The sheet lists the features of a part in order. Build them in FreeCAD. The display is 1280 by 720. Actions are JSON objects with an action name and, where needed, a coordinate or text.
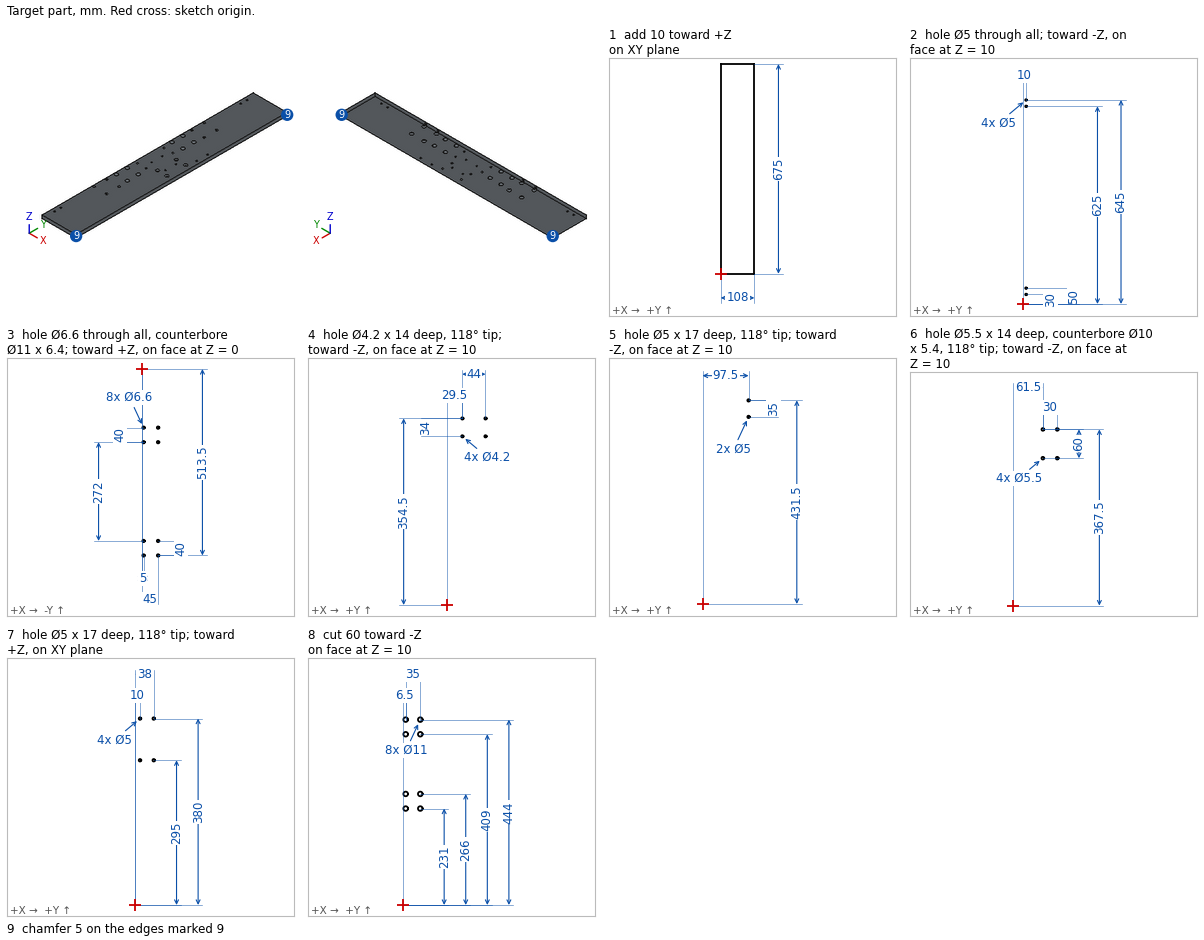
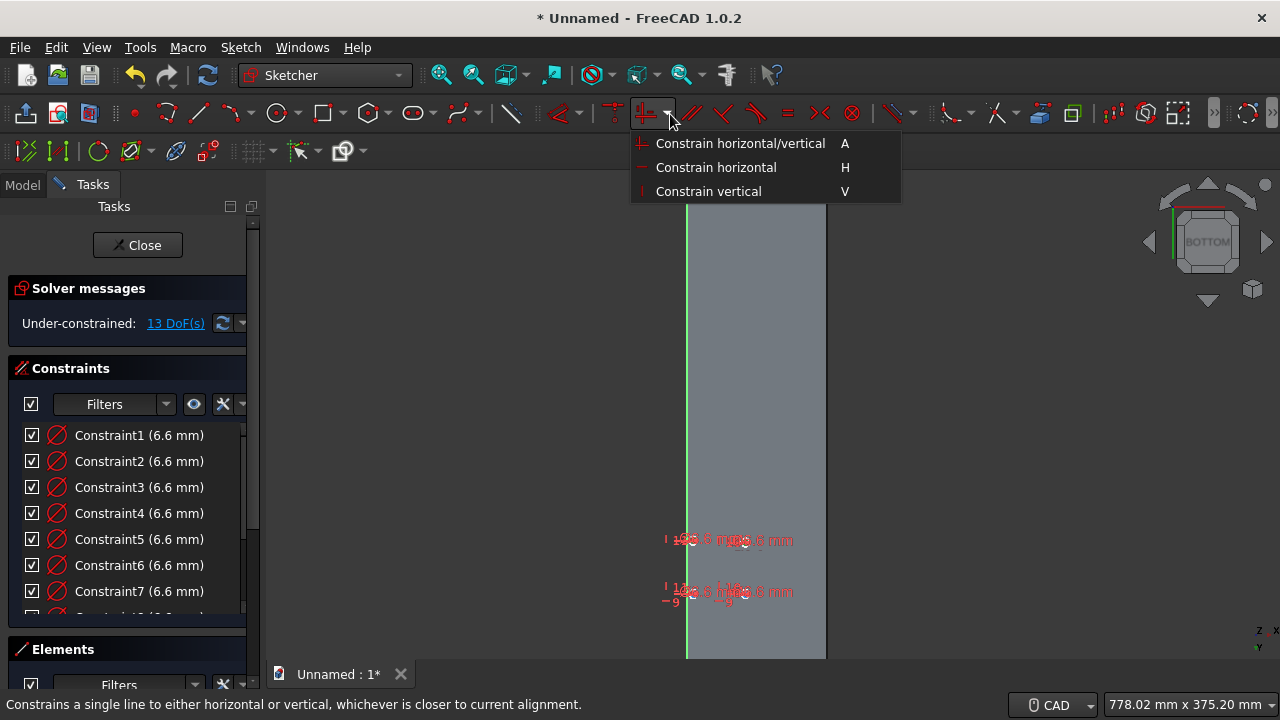
{"action": "left_click", "coordinate": [766, 167]}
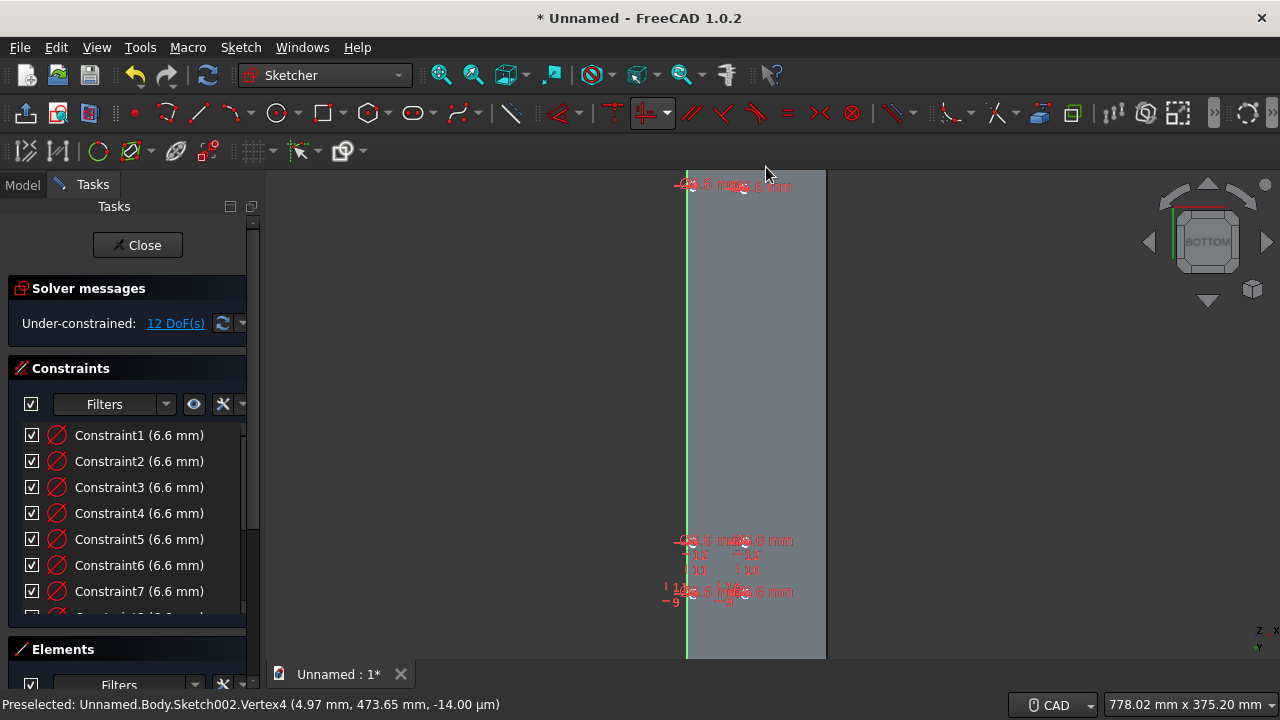
{"action": "left_click", "coordinate": [693, 543]}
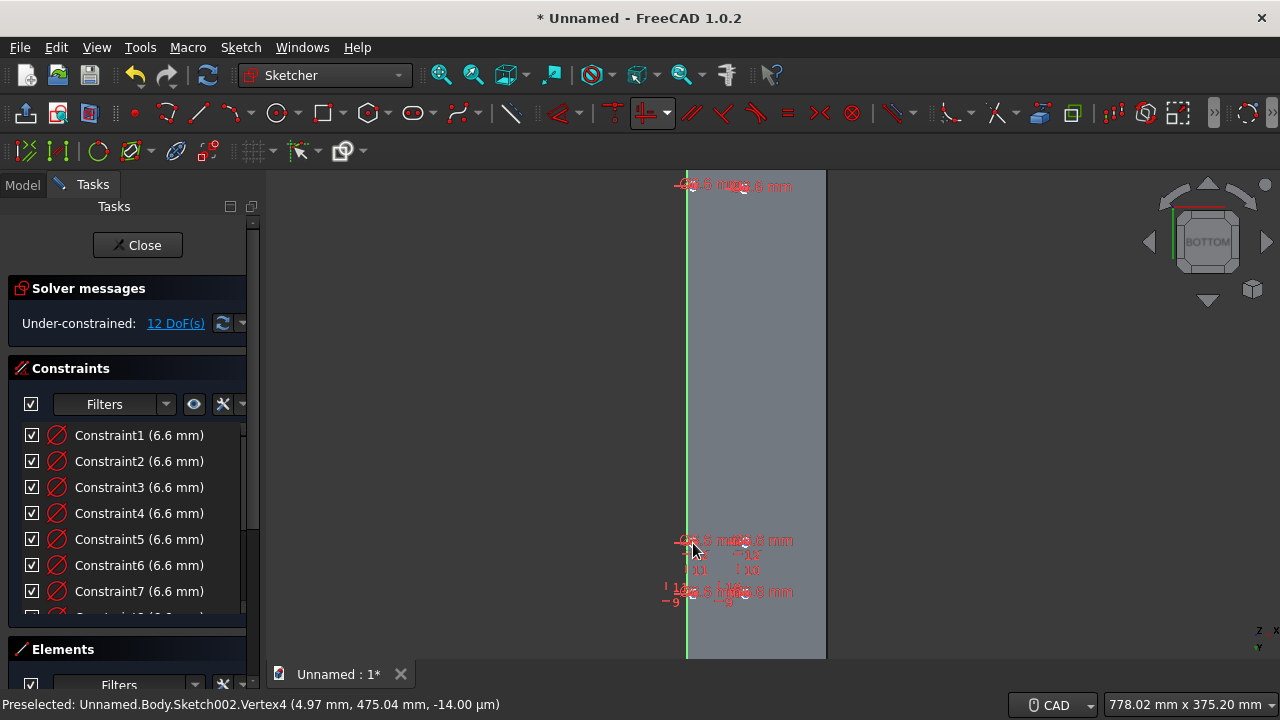
{"action": "scroll", "coordinate": [693, 540], "scroll_direction": "down", "scroll_amount": 4}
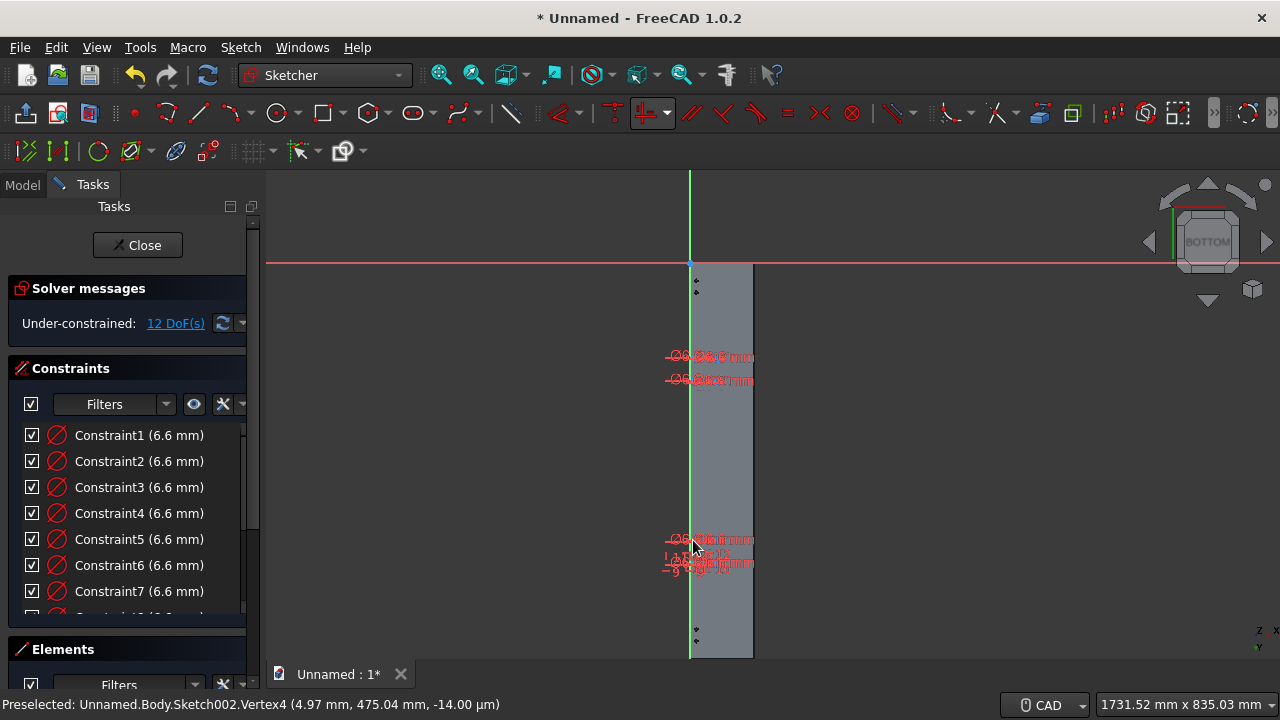
{"action": "left_click", "coordinate": [693, 381]}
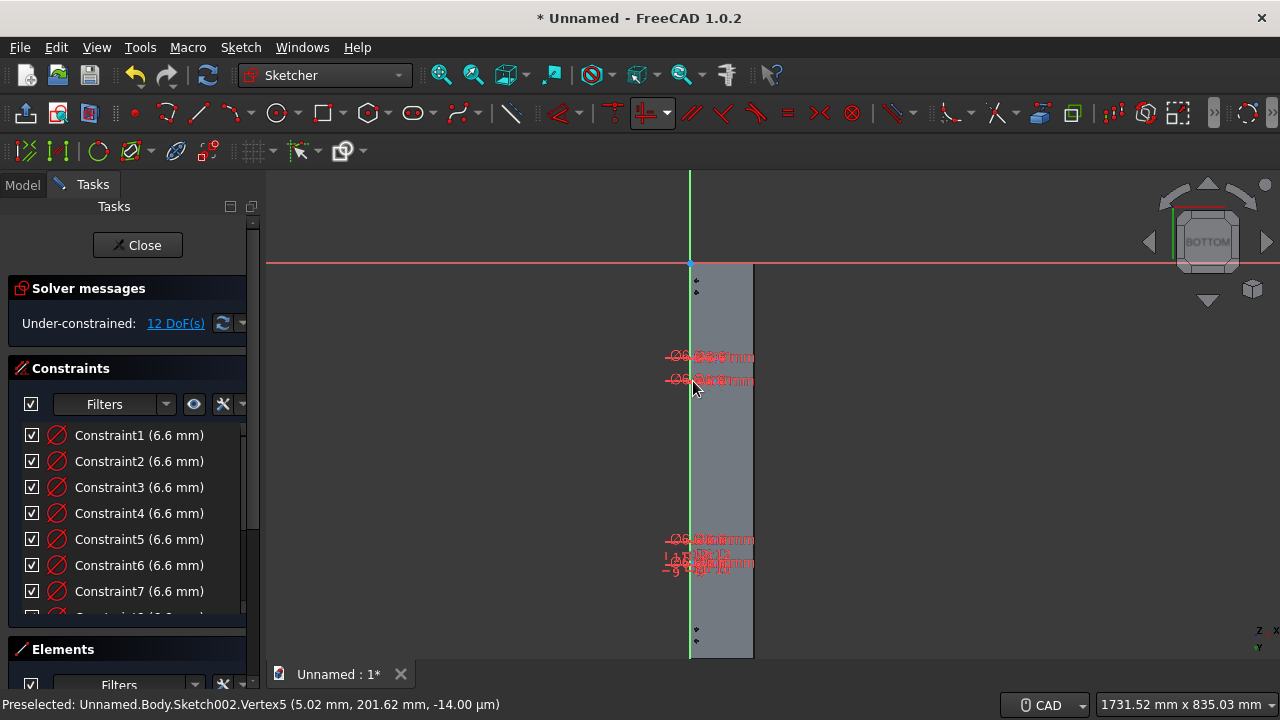
{"action": "key", "text": "v"}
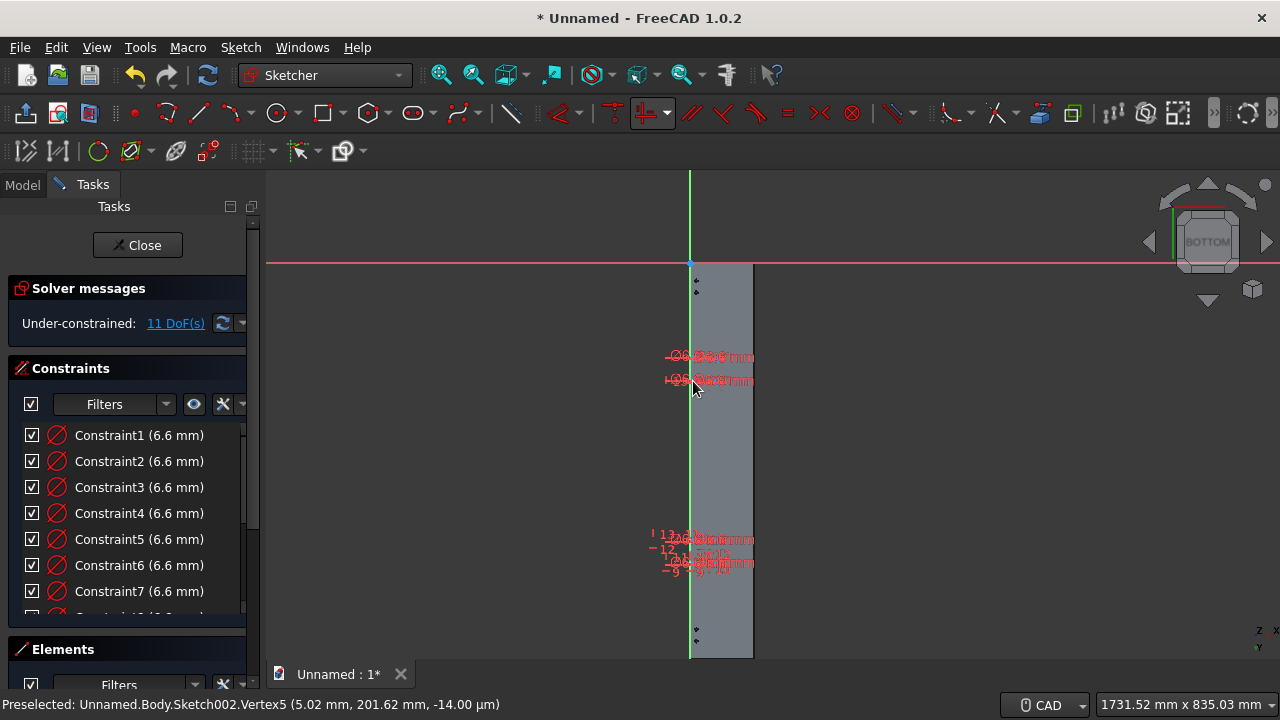
{"action": "left_click", "coordinate": [717, 542]}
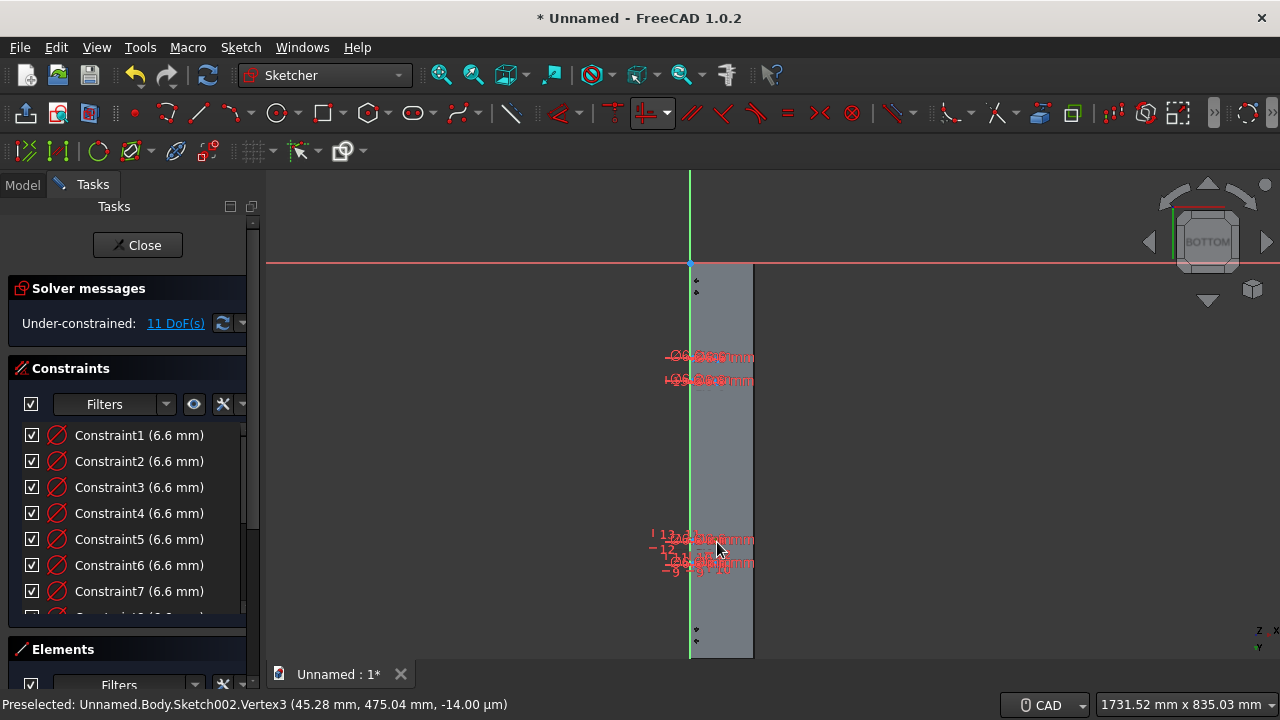
{"action": "left_click", "coordinate": [716, 383]}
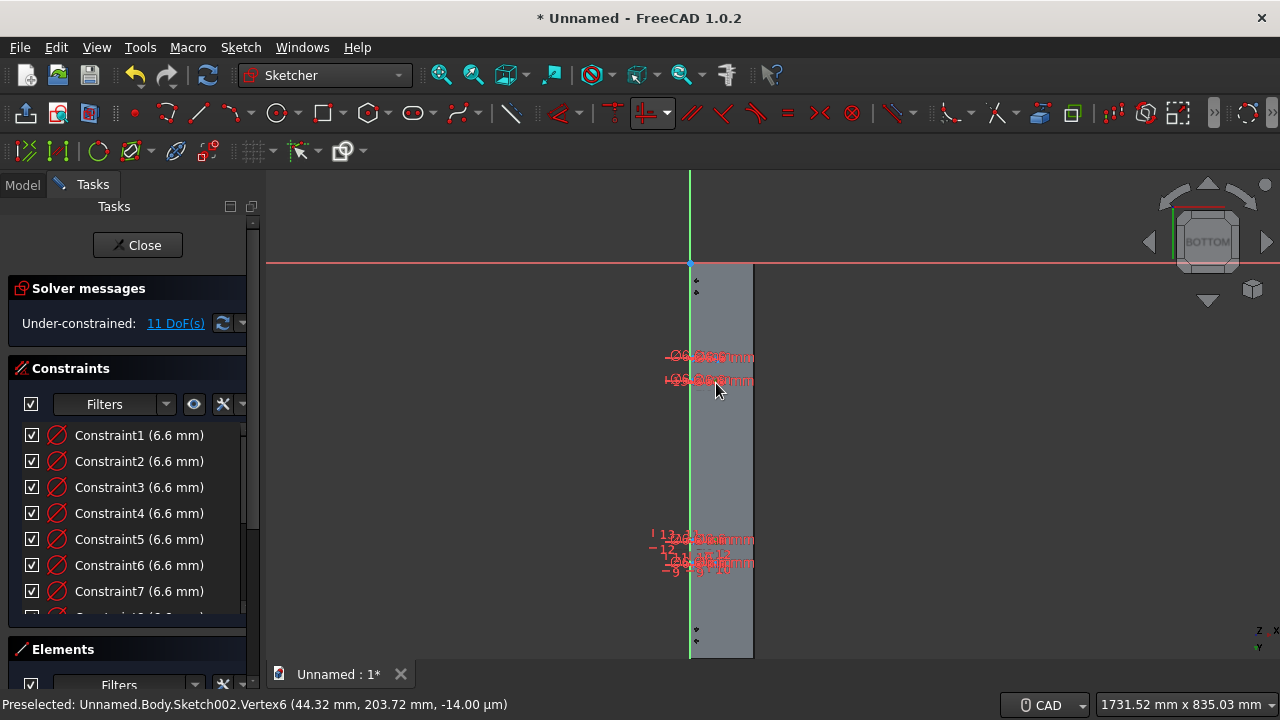
{"action": "key", "text": "v"}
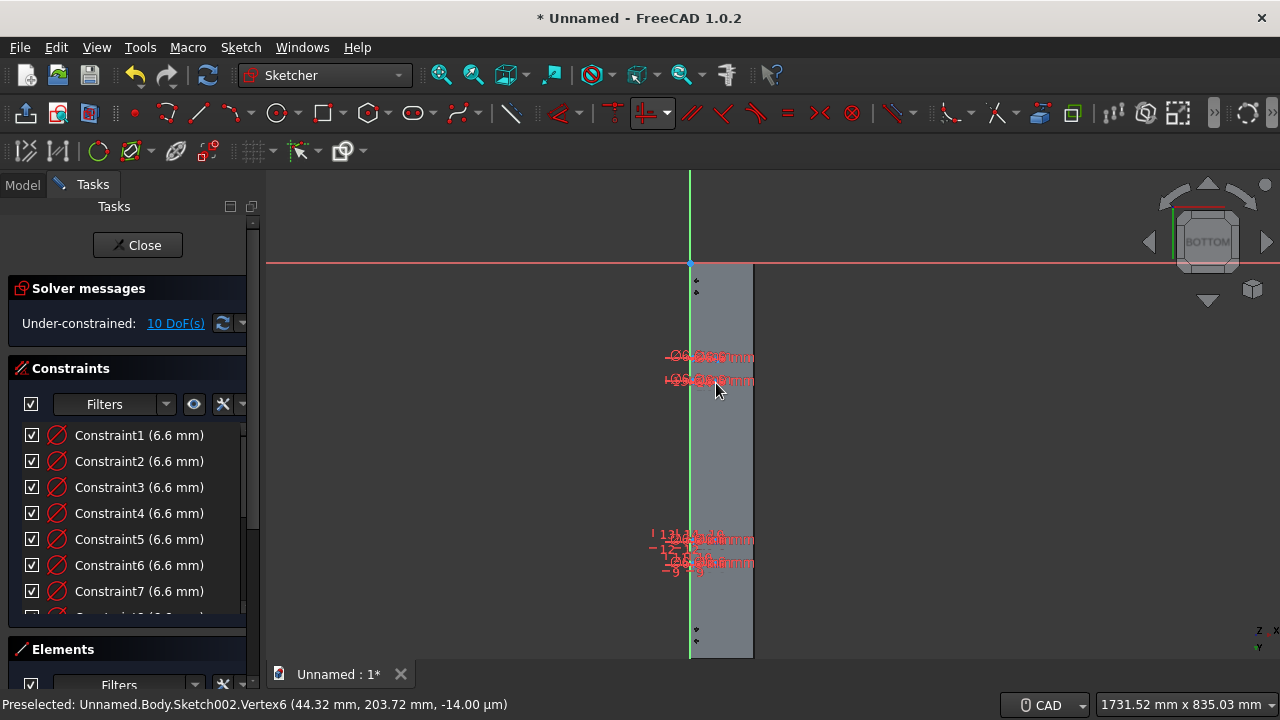
{"action": "scroll", "coordinate": [693, 381], "scroll_direction": "up", "scroll_amount": 4}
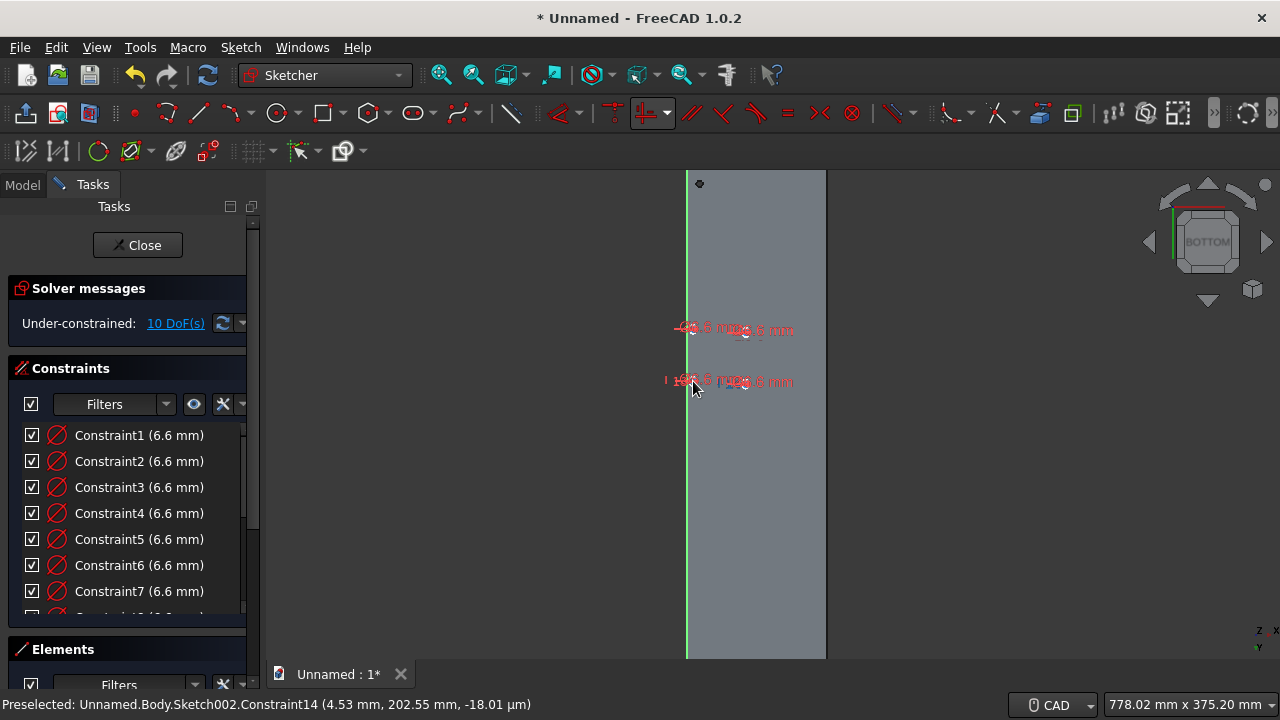
{"action": "left_click", "coordinate": [693, 381]}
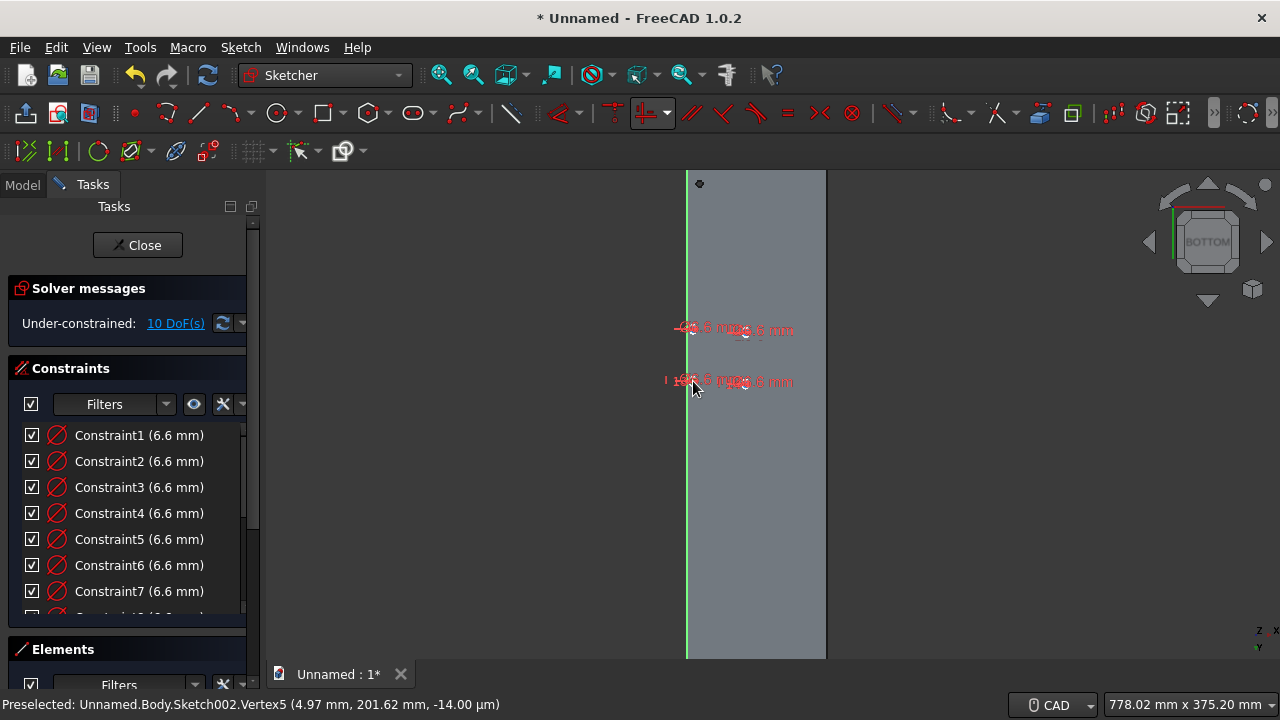
{"action": "left_click", "coordinate": [746, 384]}